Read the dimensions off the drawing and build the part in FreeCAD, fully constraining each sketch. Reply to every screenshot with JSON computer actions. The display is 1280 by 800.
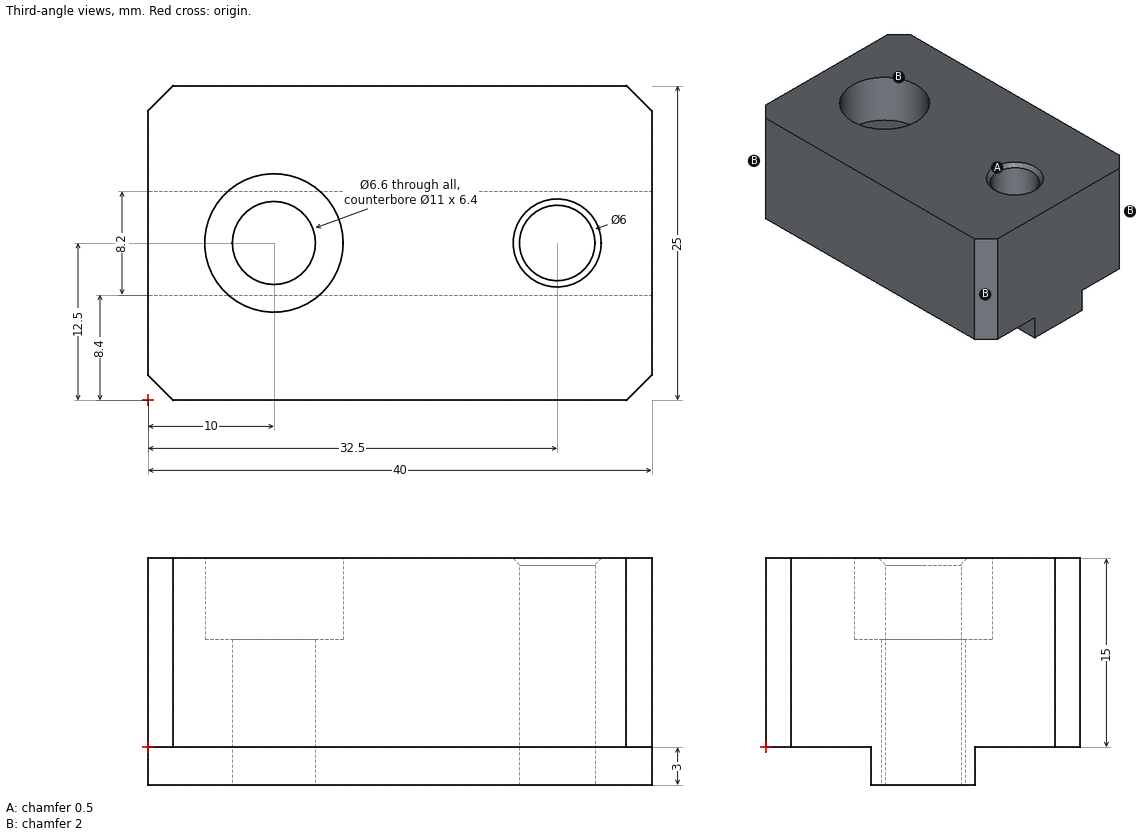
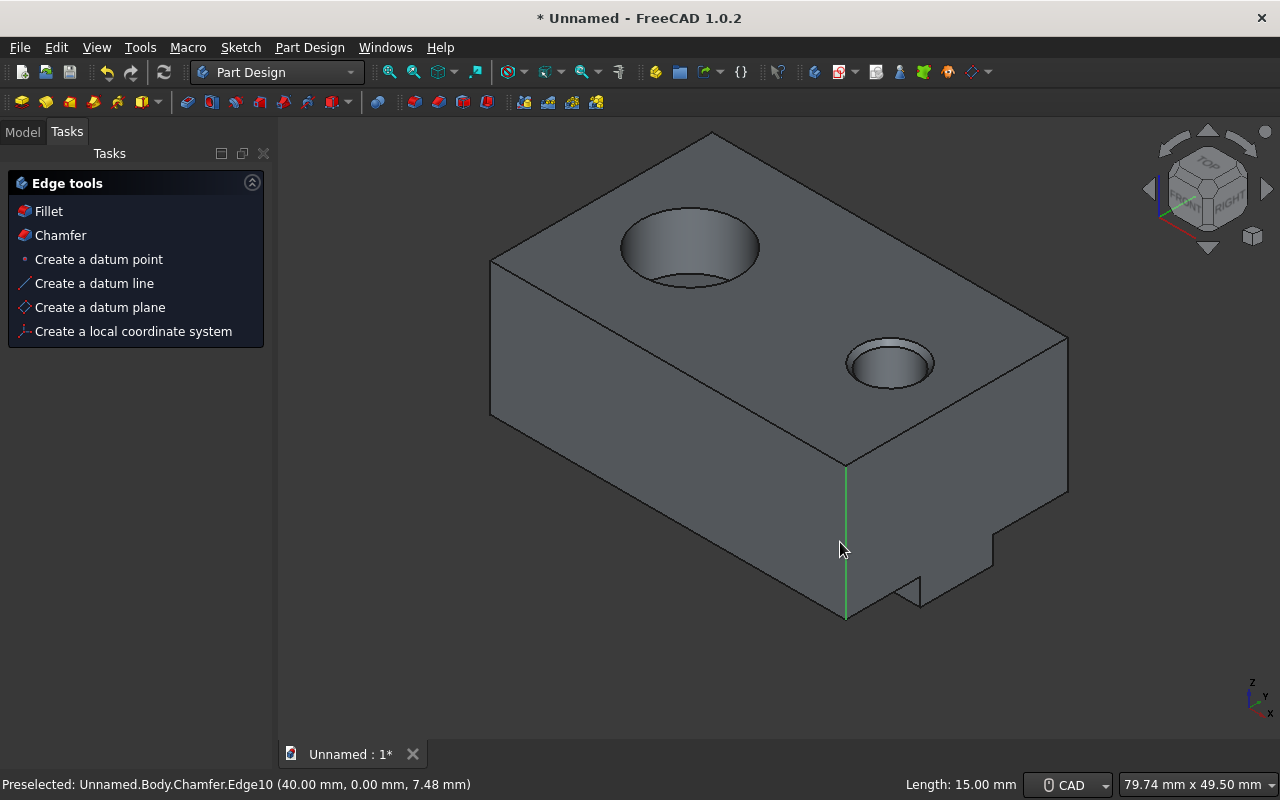
{"action": "key", "text": "2"}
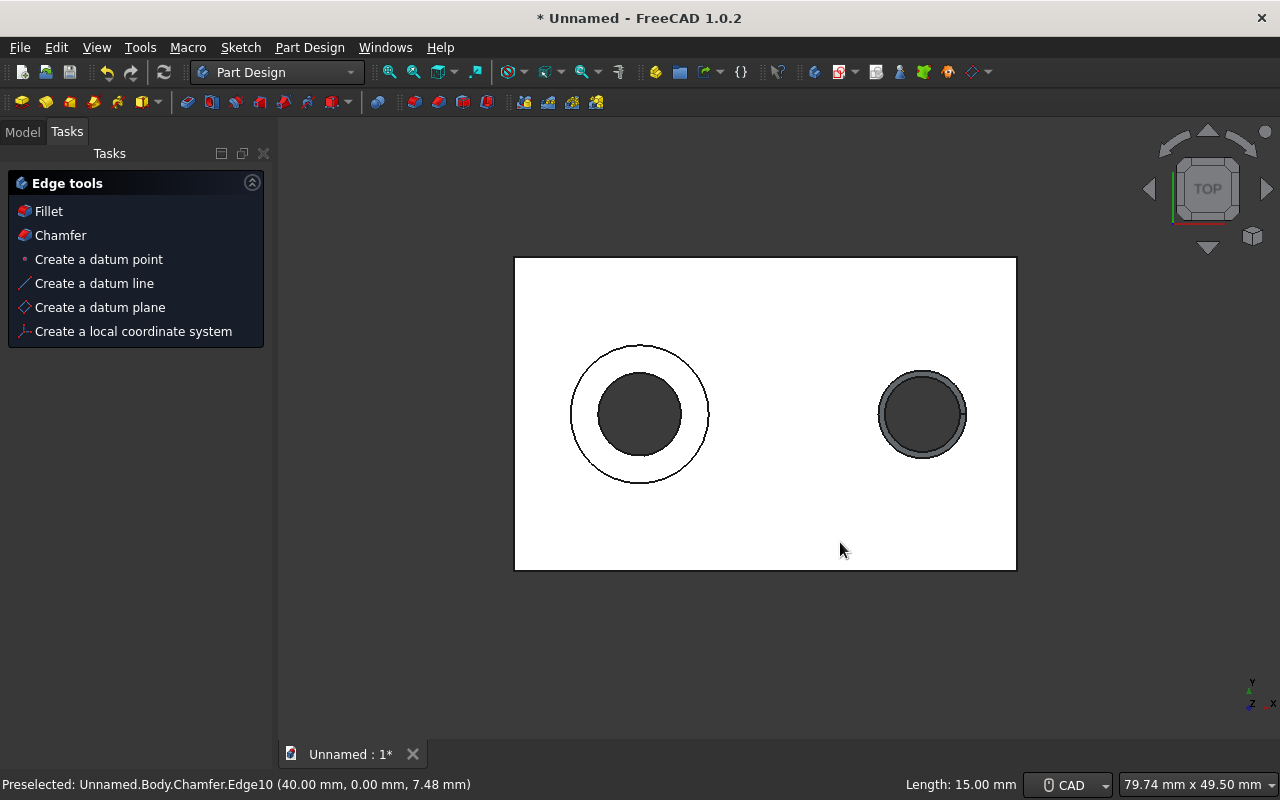
{"action": "key", "text": "0"}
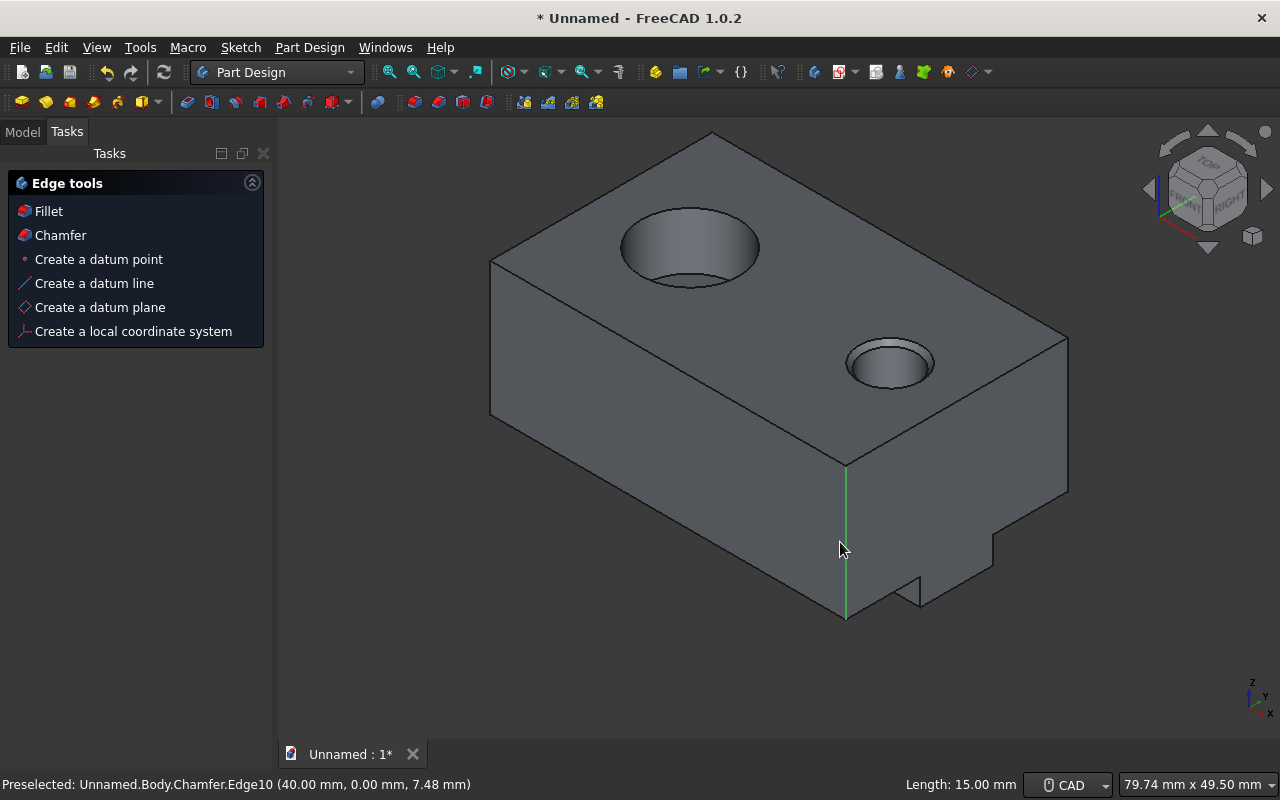
{"action": "key", "text": "1"}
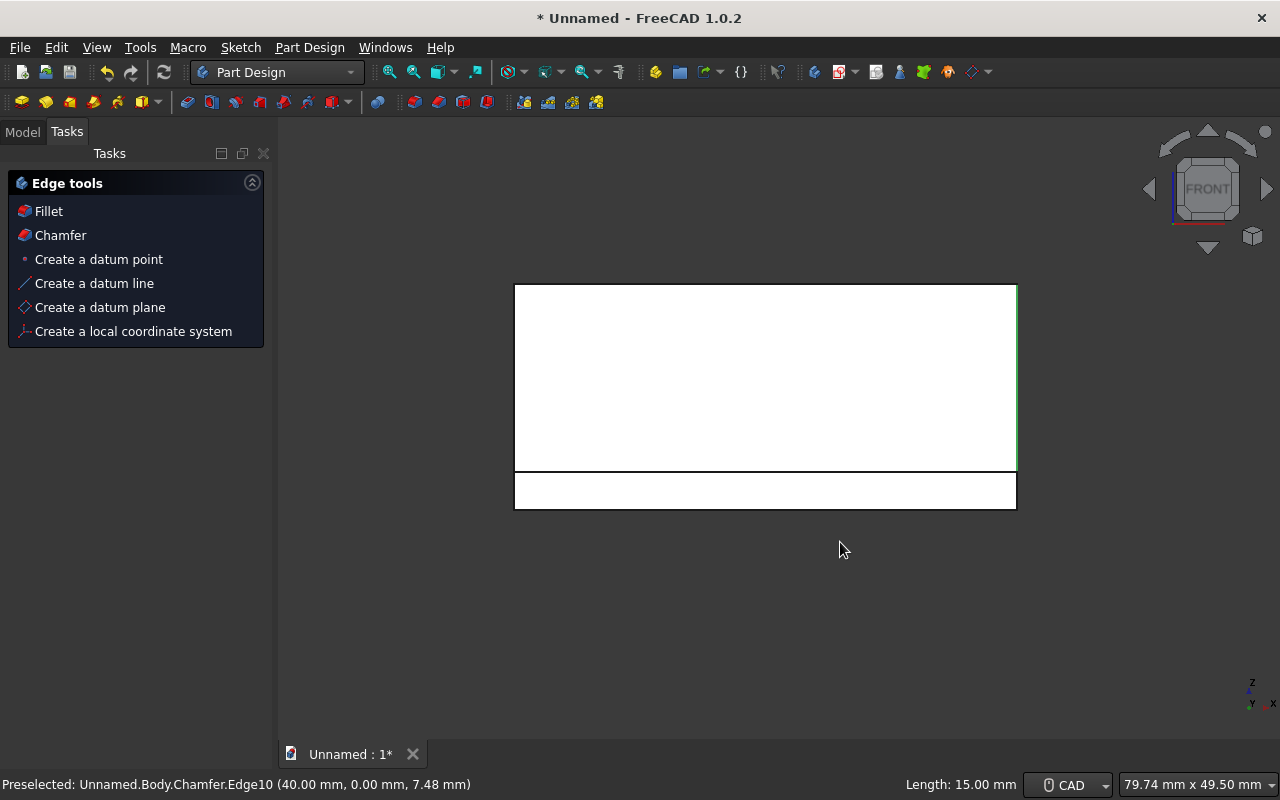
{"action": "left_click", "coordinate": [514, 377], "text": "ctrl"}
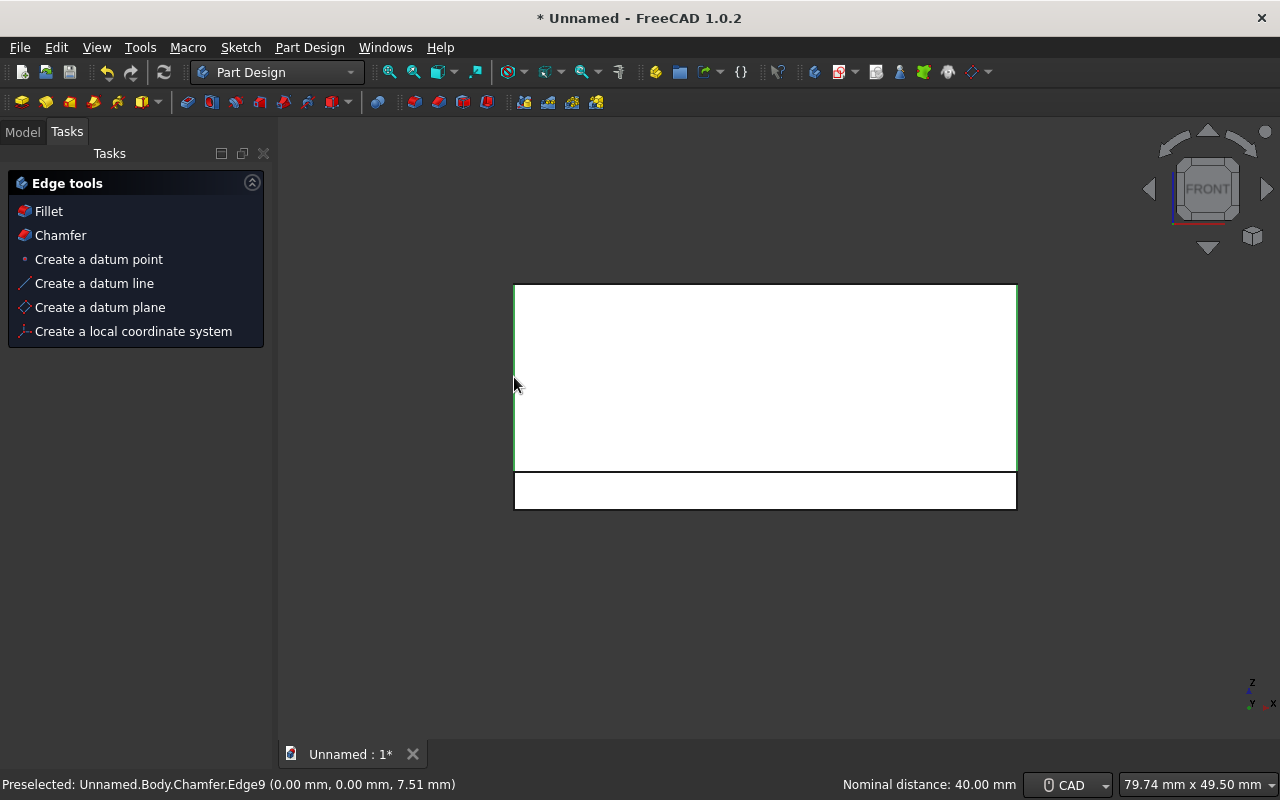
{"action": "key", "text": "3"}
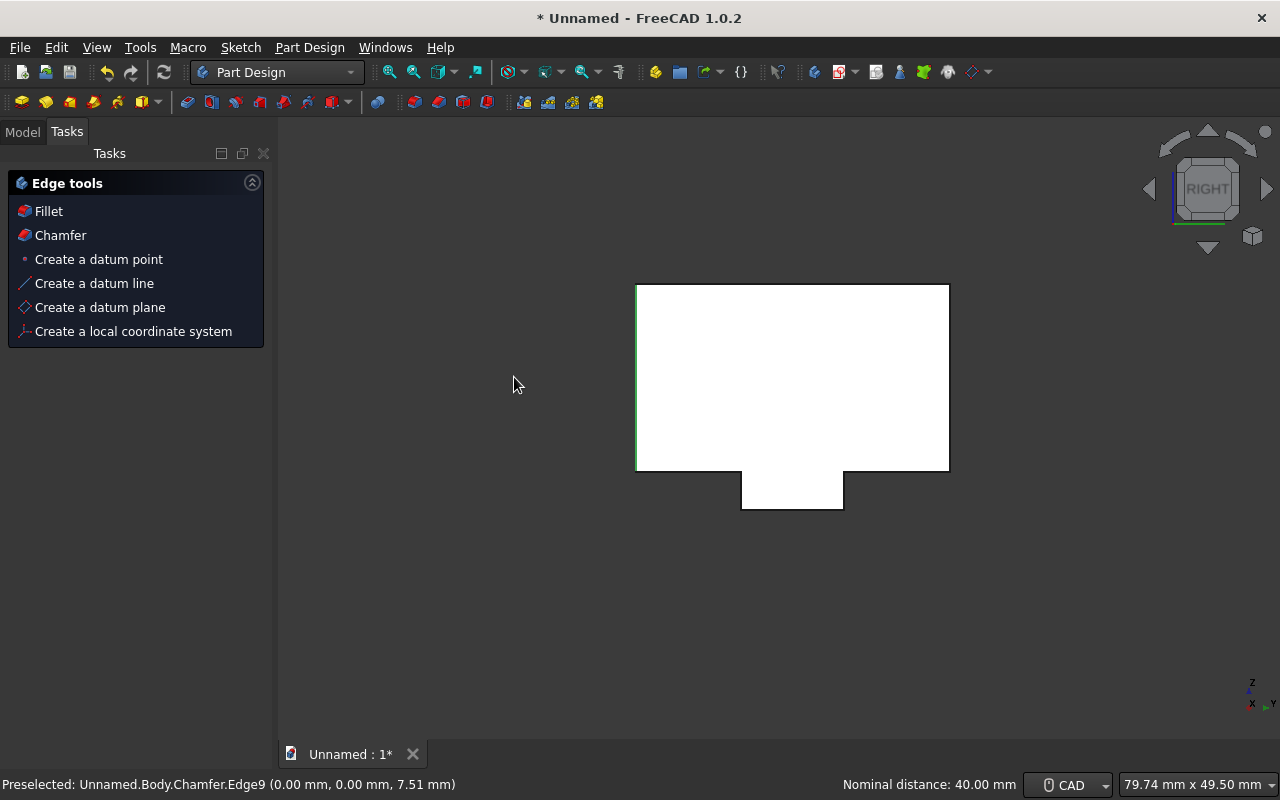
{"action": "left_click", "coordinate": [390, 72]}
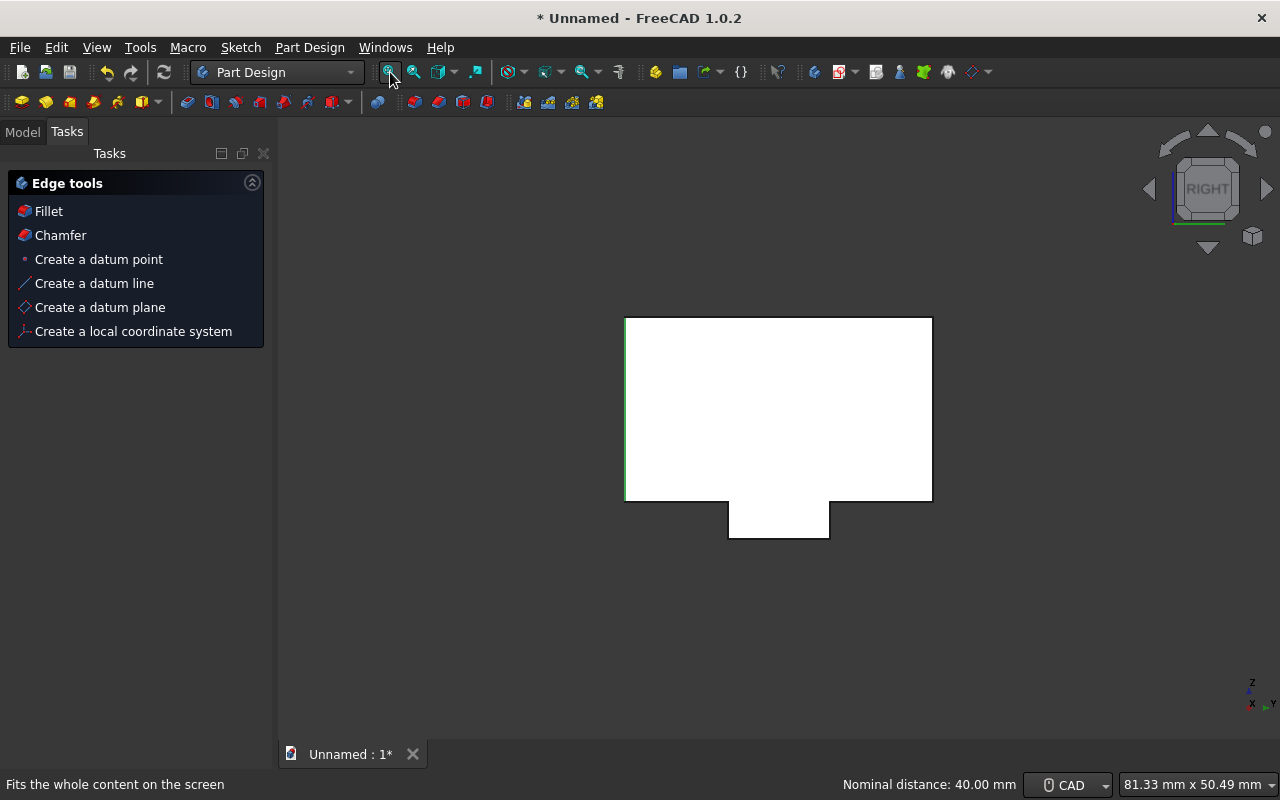
{"action": "left_click", "coordinate": [933, 409], "text": "ctrl"}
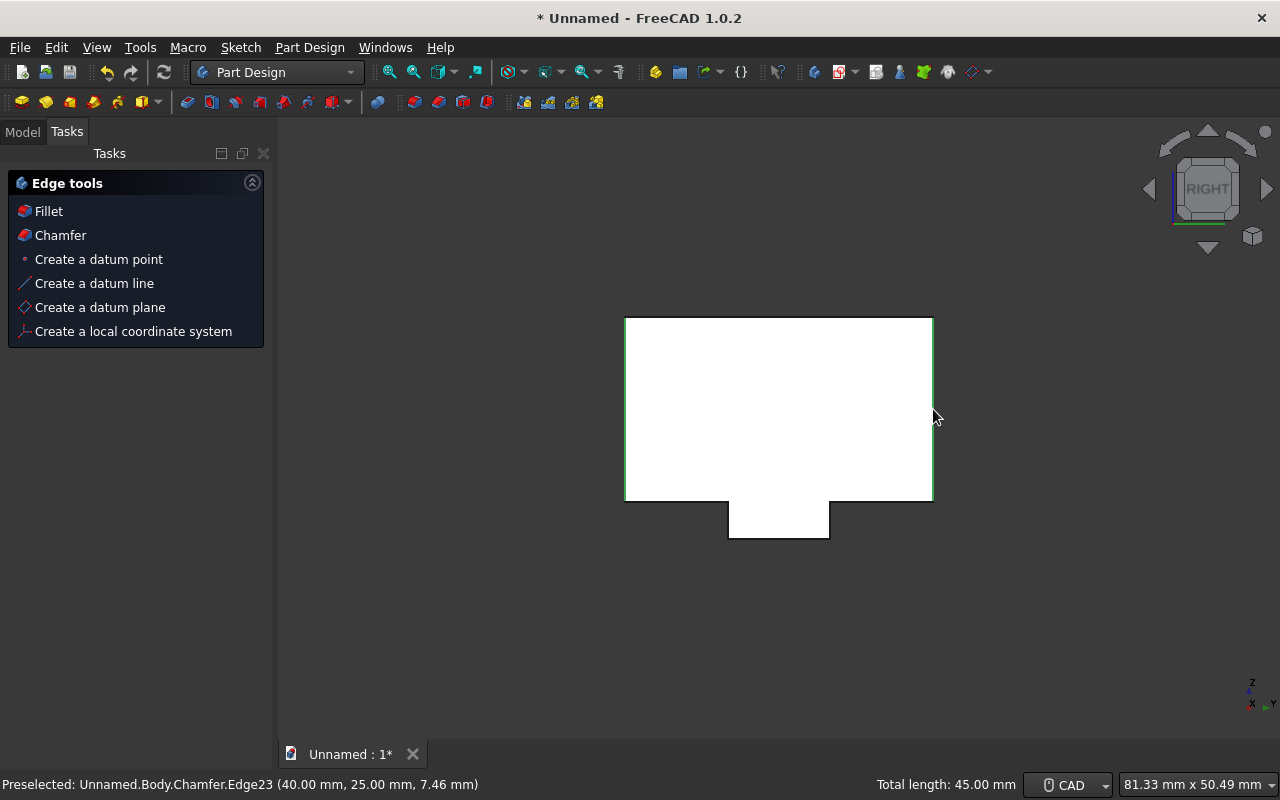
{"action": "key", "text": "5"}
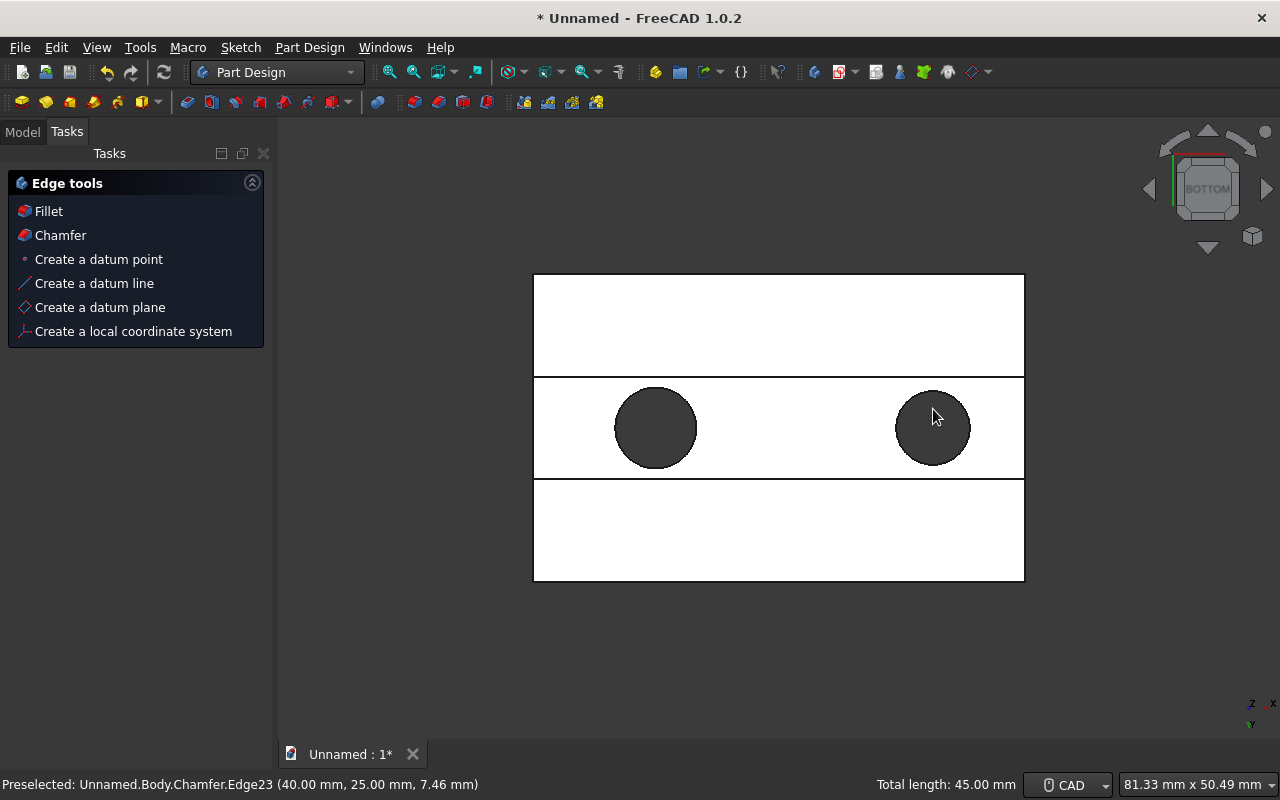
{"action": "key", "text": "4"}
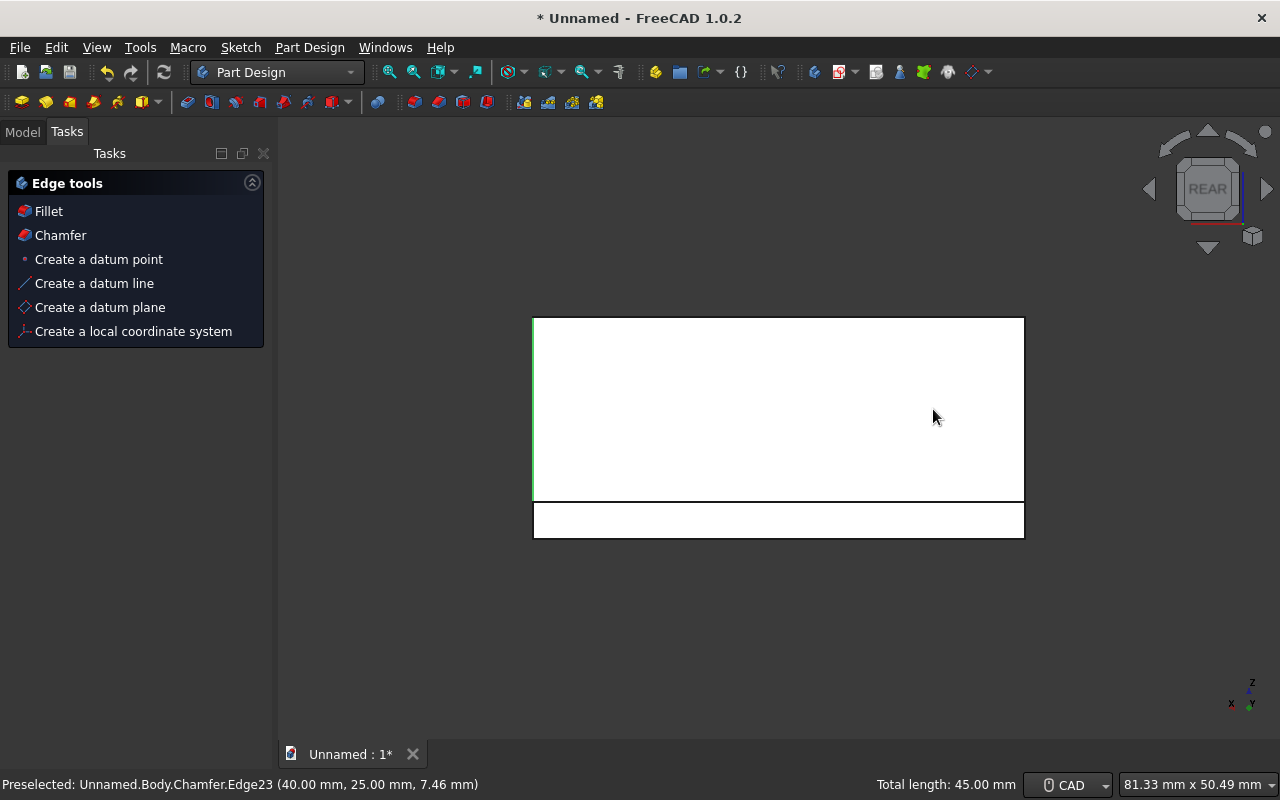
{"action": "left_click", "coordinate": [1025, 409], "text": "ctrl"}